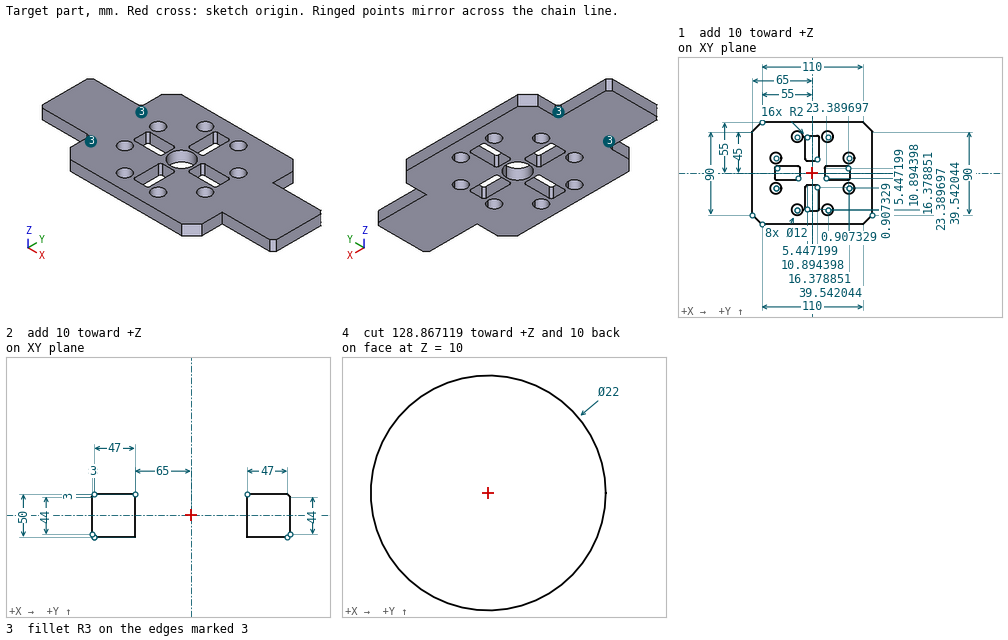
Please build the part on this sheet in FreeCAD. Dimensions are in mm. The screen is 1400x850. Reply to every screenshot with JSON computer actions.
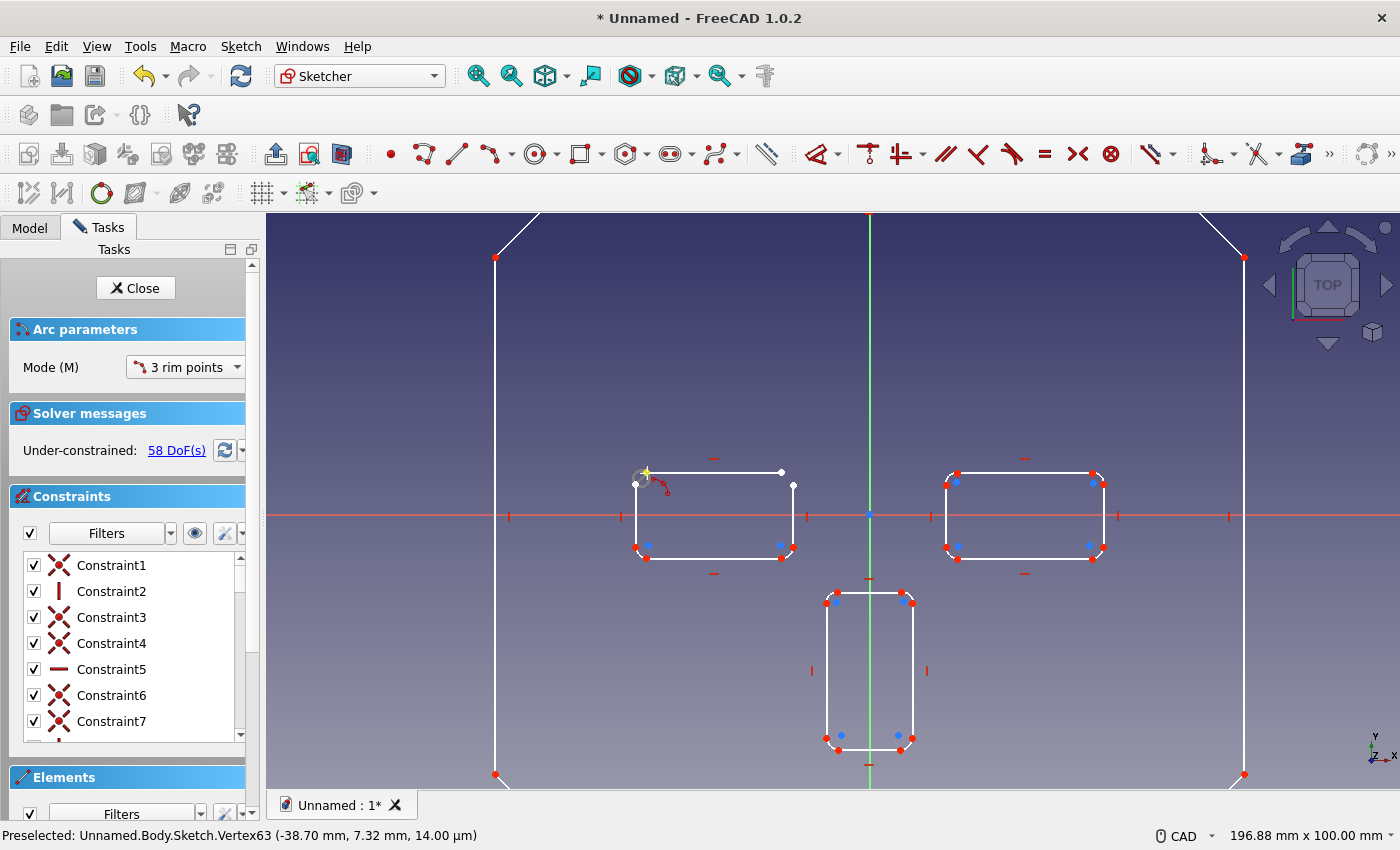
{"action": "scroll", "coordinate": [639, 475], "scroll_direction": "up", "scroll_amount": 8}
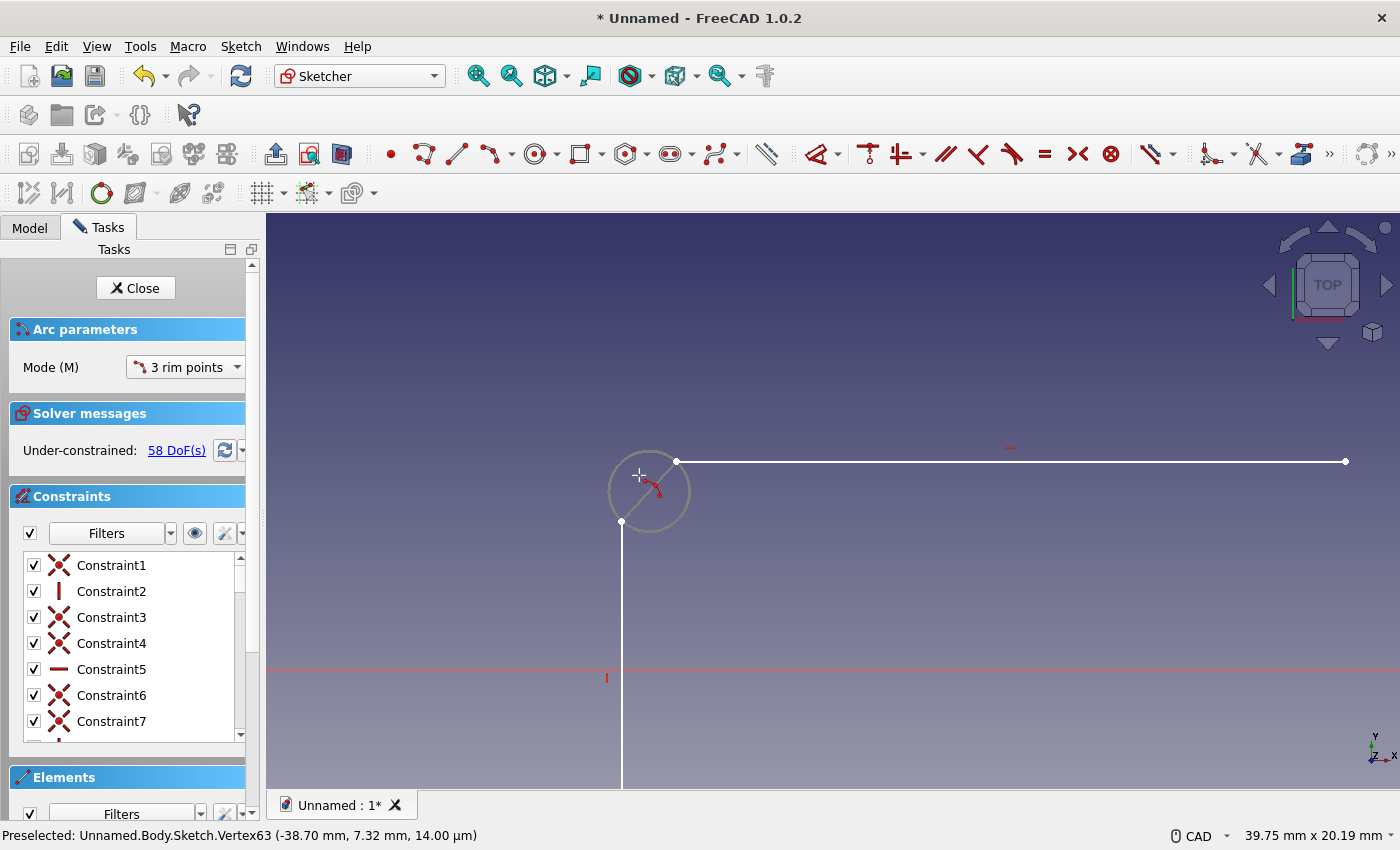
{"action": "left_click", "coordinate": [638, 475]}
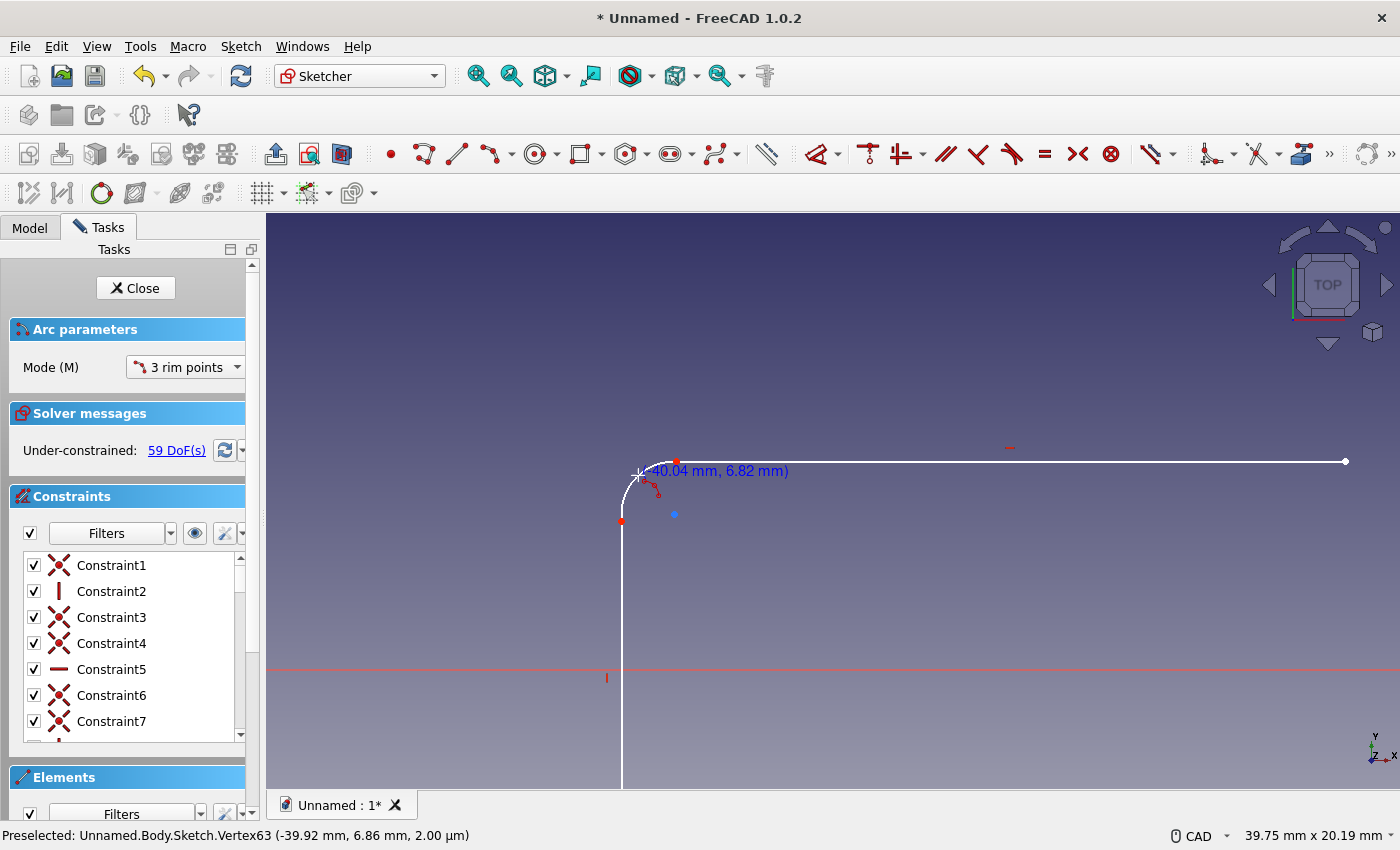
{"action": "scroll", "coordinate": [638, 480], "scroll_direction": "down", "scroll_amount": 11}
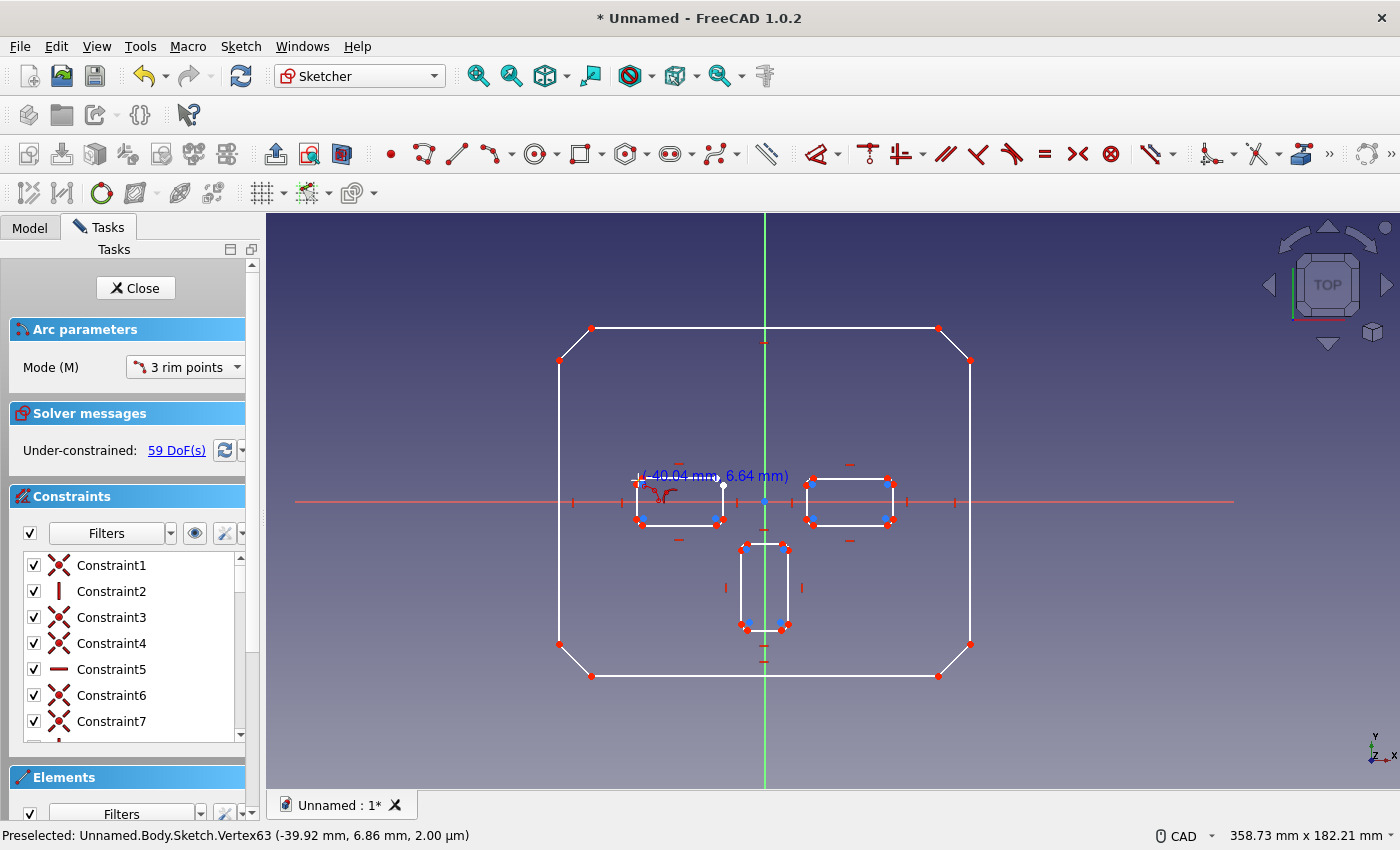
{"action": "scroll", "coordinate": [717, 478], "scroll_direction": "up", "scroll_amount": 3}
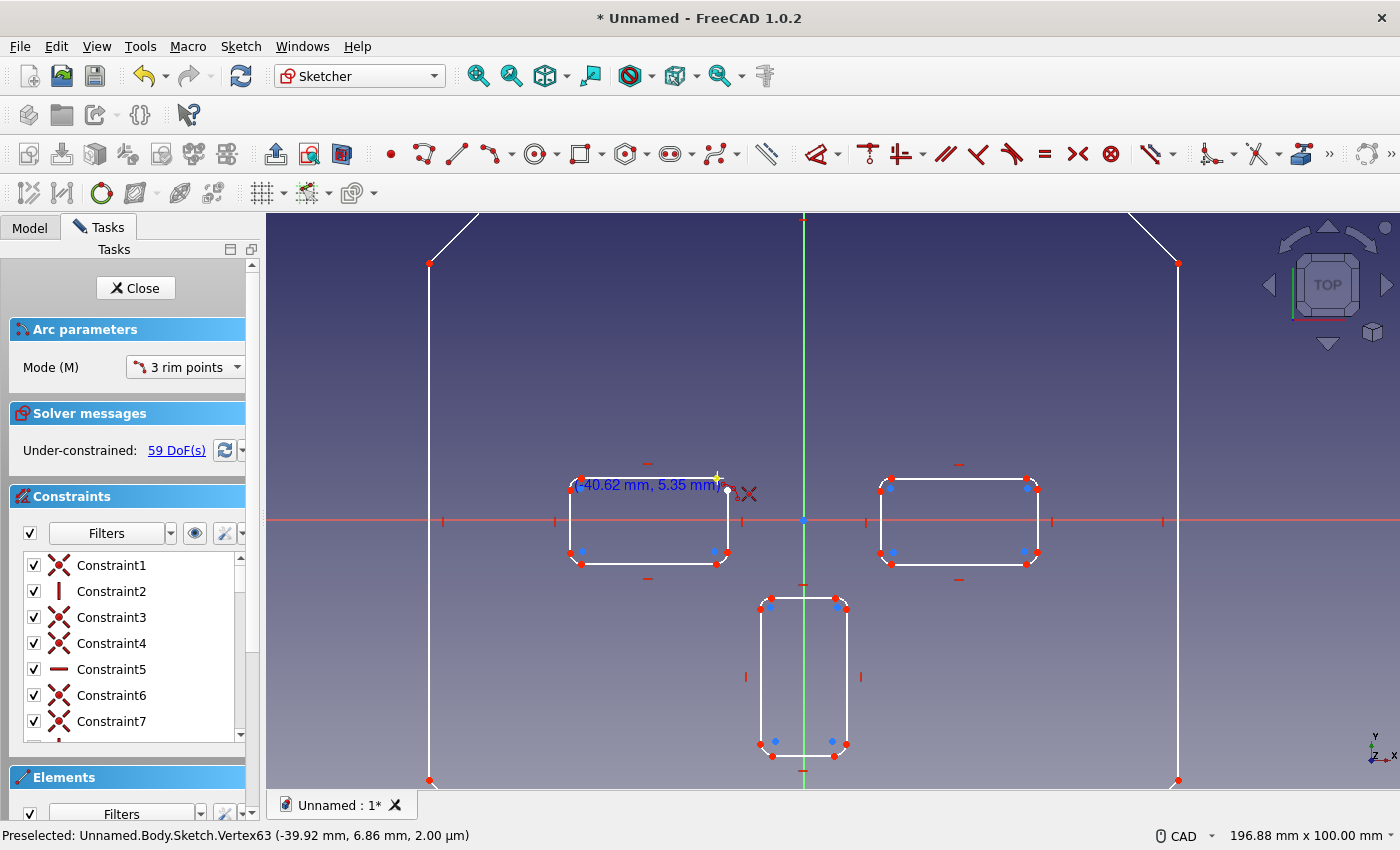
{"action": "left_click", "coordinate": [716, 478]}
{"action": "left_click", "coordinate": [728, 491]}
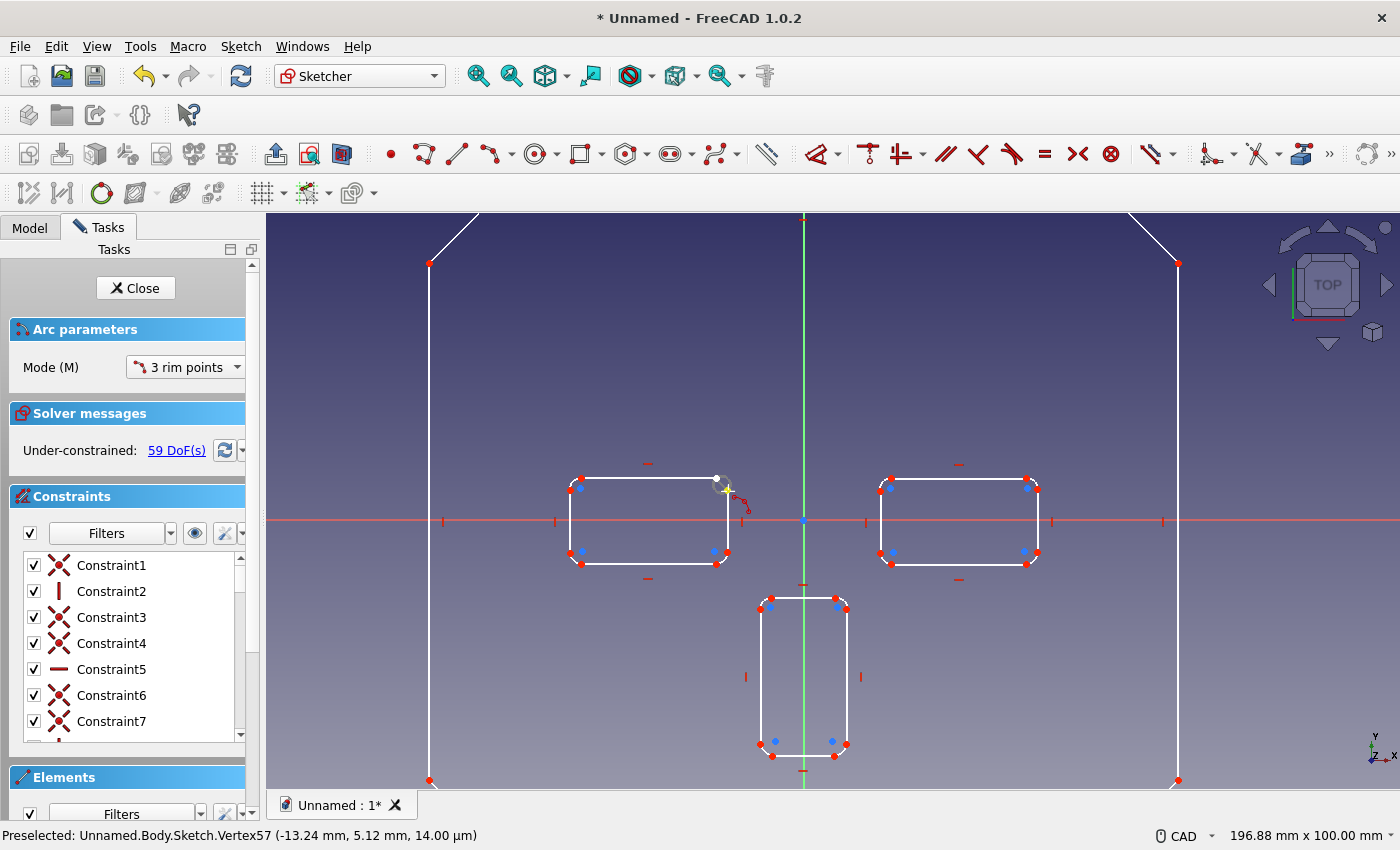
{"action": "scroll", "coordinate": [724, 481], "scroll_direction": "up", "scroll_amount": 8}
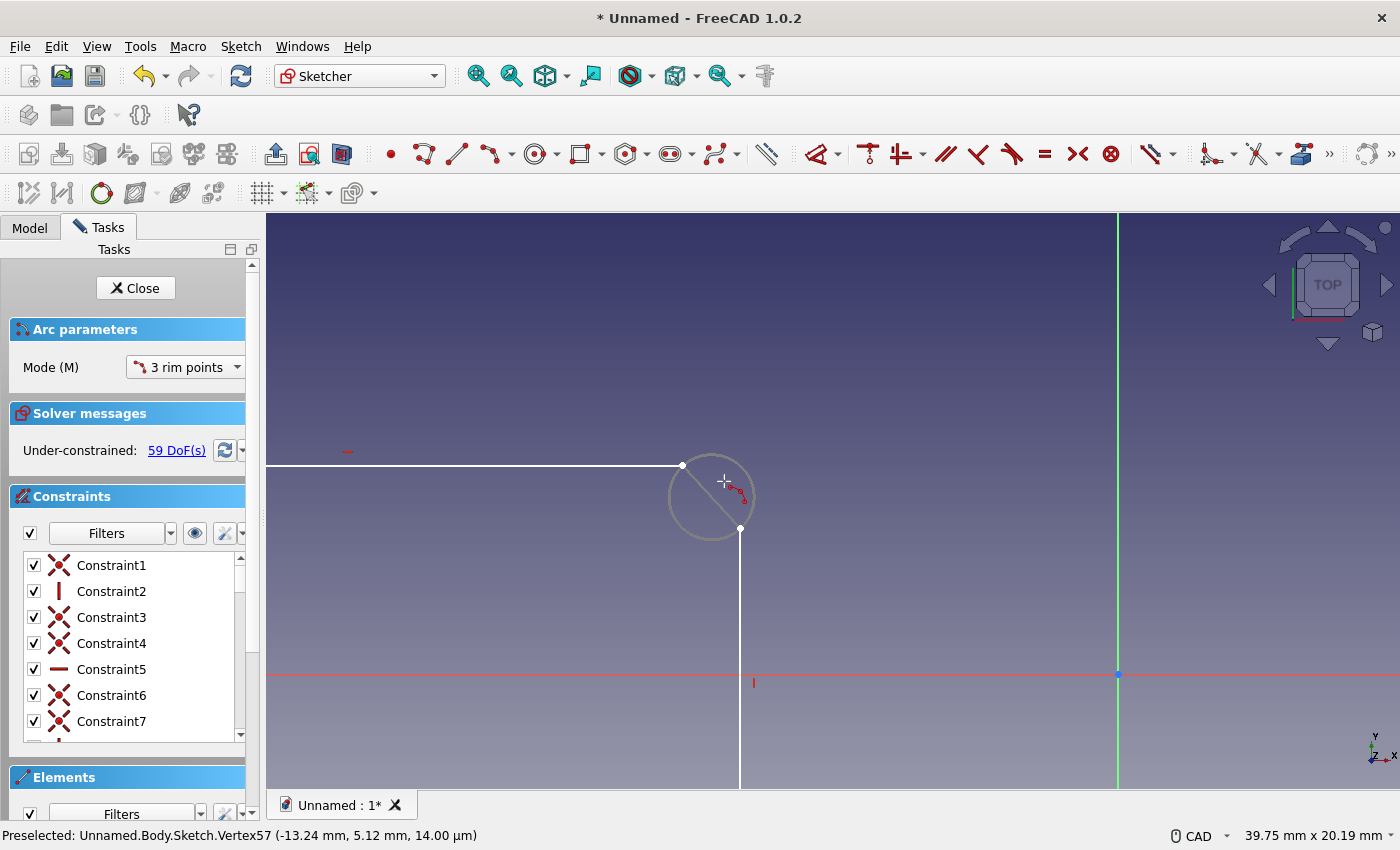
{"action": "left_click", "coordinate": [724, 479]}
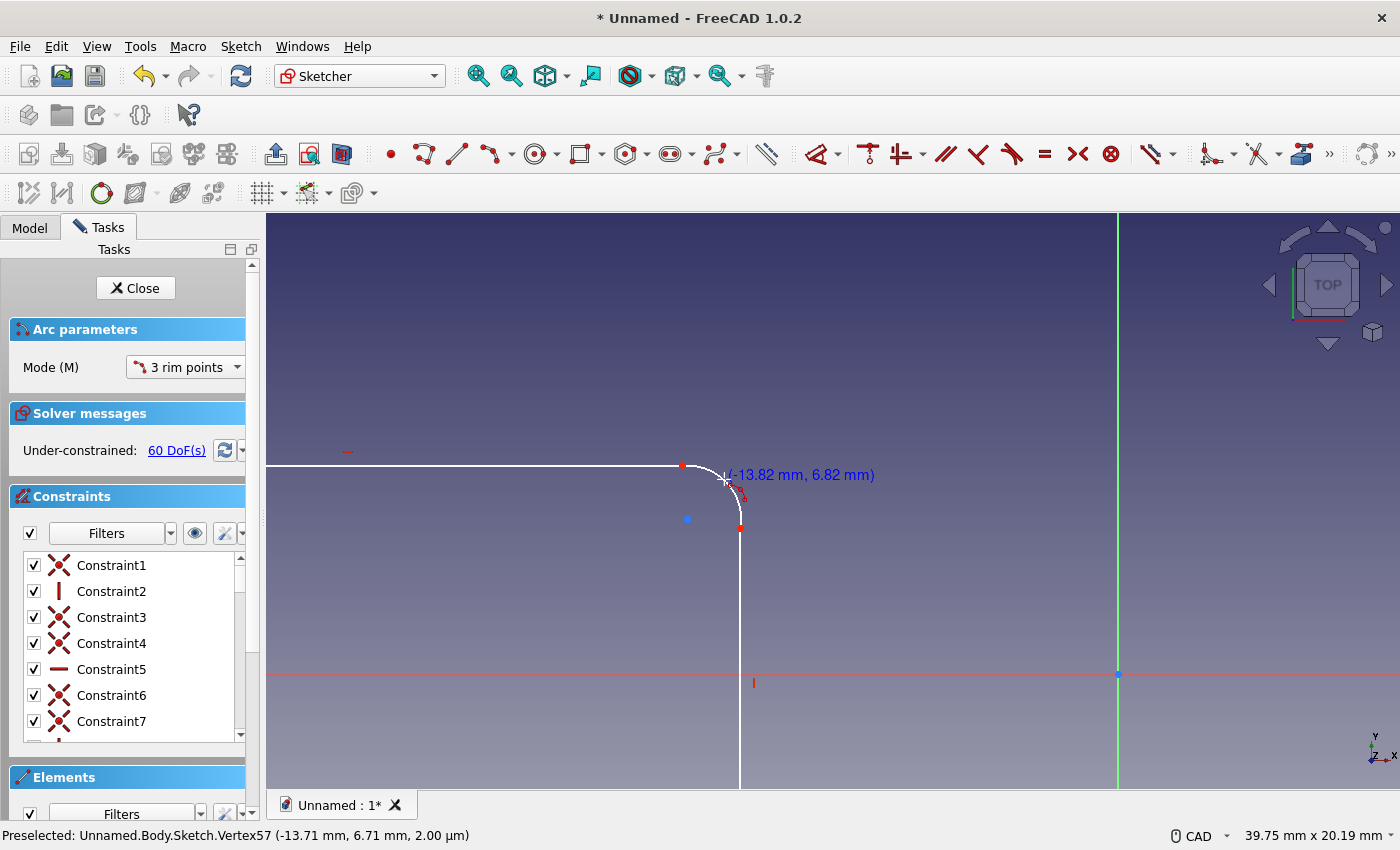
{"action": "left_click", "coordinate": [457, 154]}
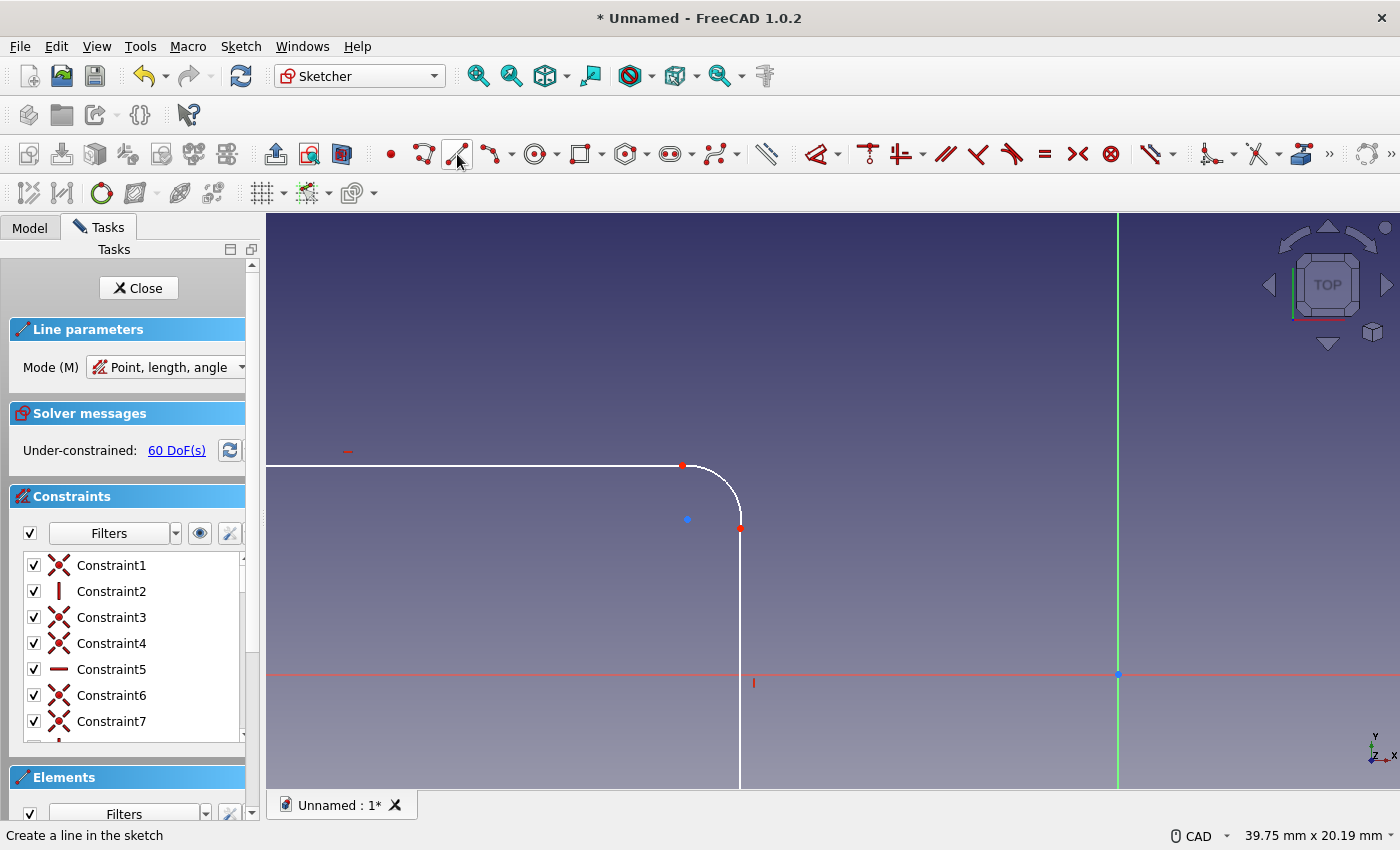
{"action": "scroll", "coordinate": [720, 479], "scroll_direction": "down", "scroll_amount": 11}